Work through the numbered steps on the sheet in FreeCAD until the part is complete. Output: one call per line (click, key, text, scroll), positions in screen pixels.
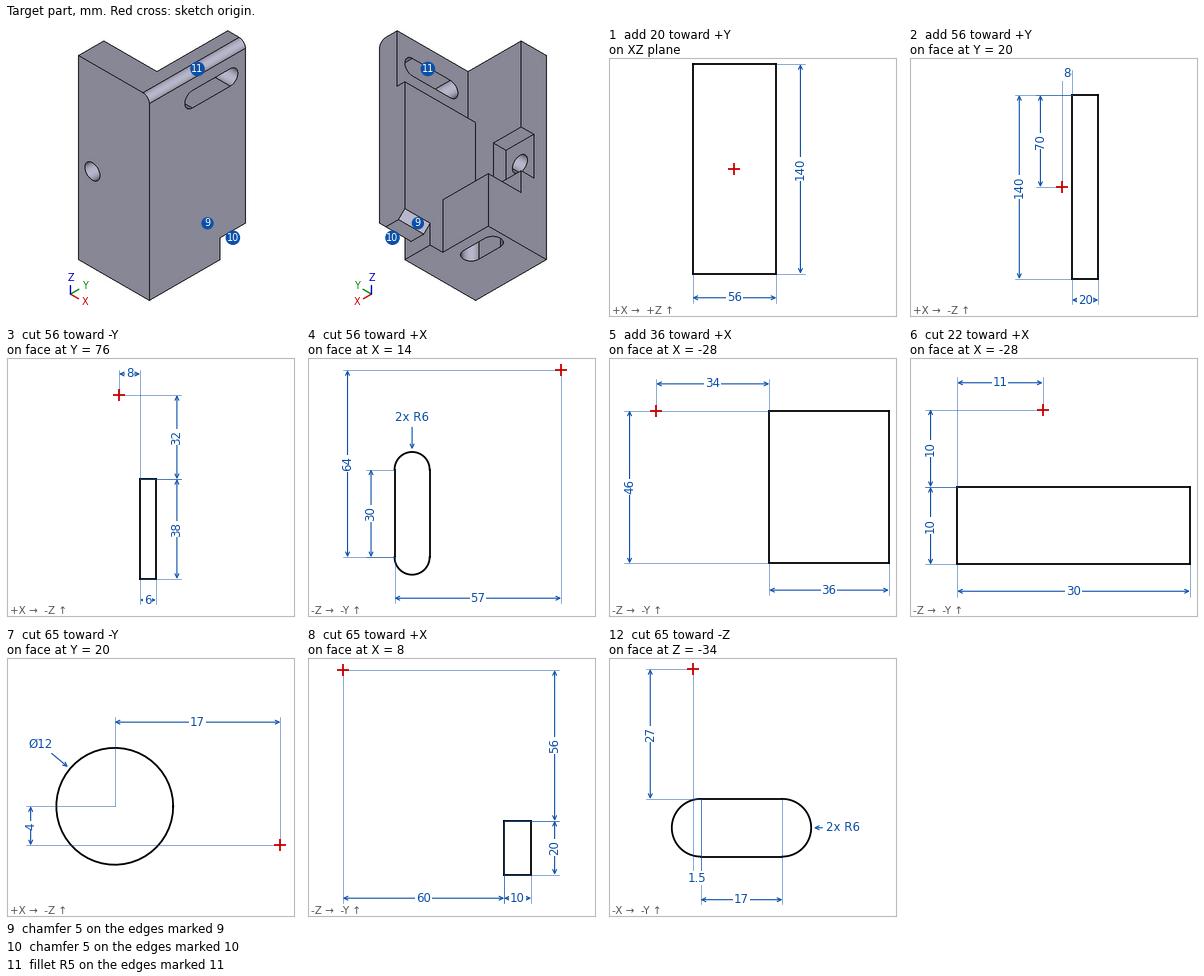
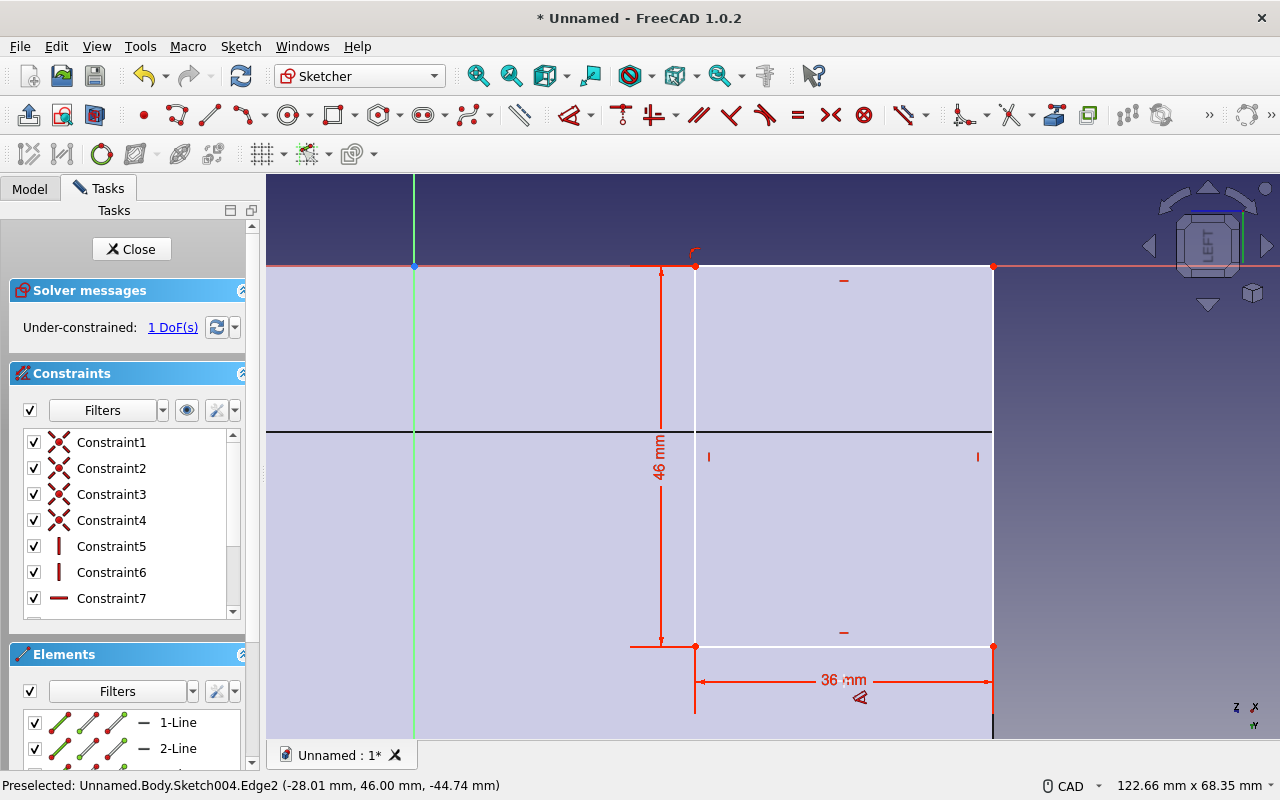
click(695, 266)
click(555, 232)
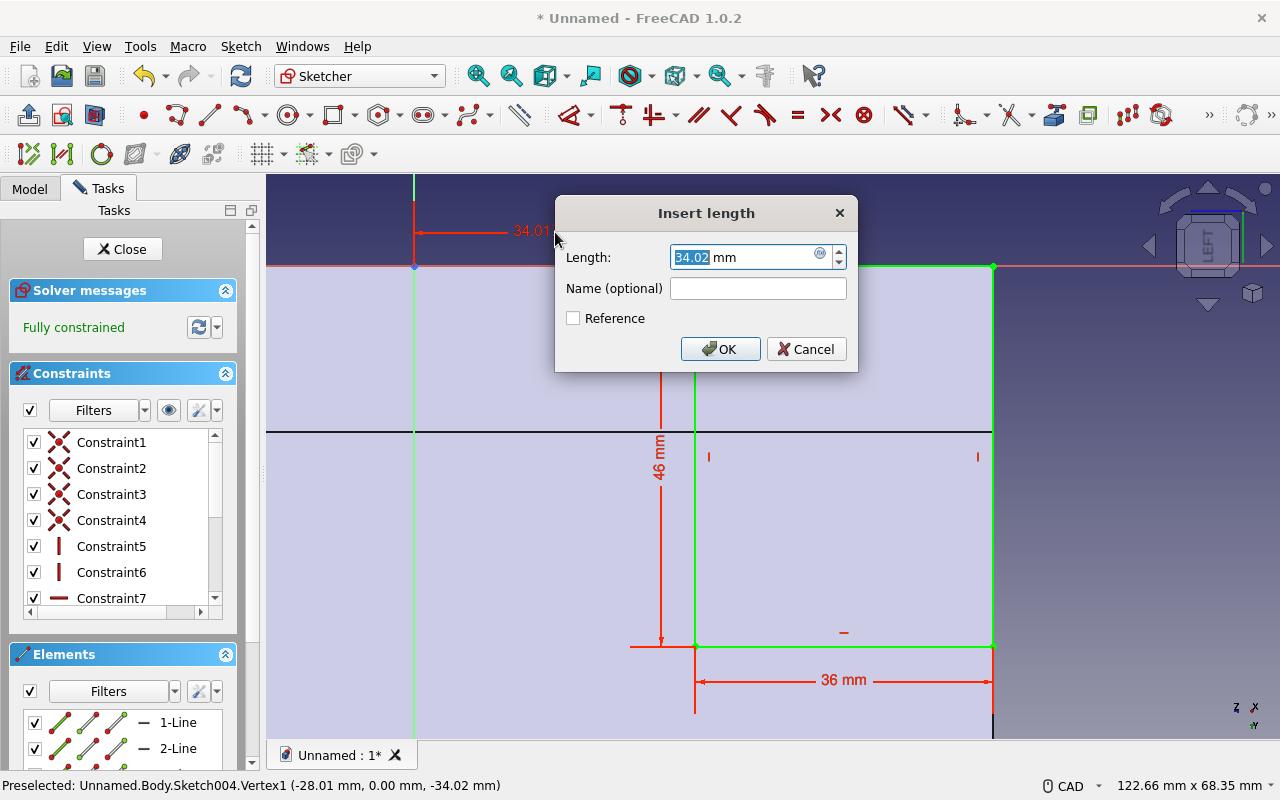
text(34)
key(Return)
key(Escape)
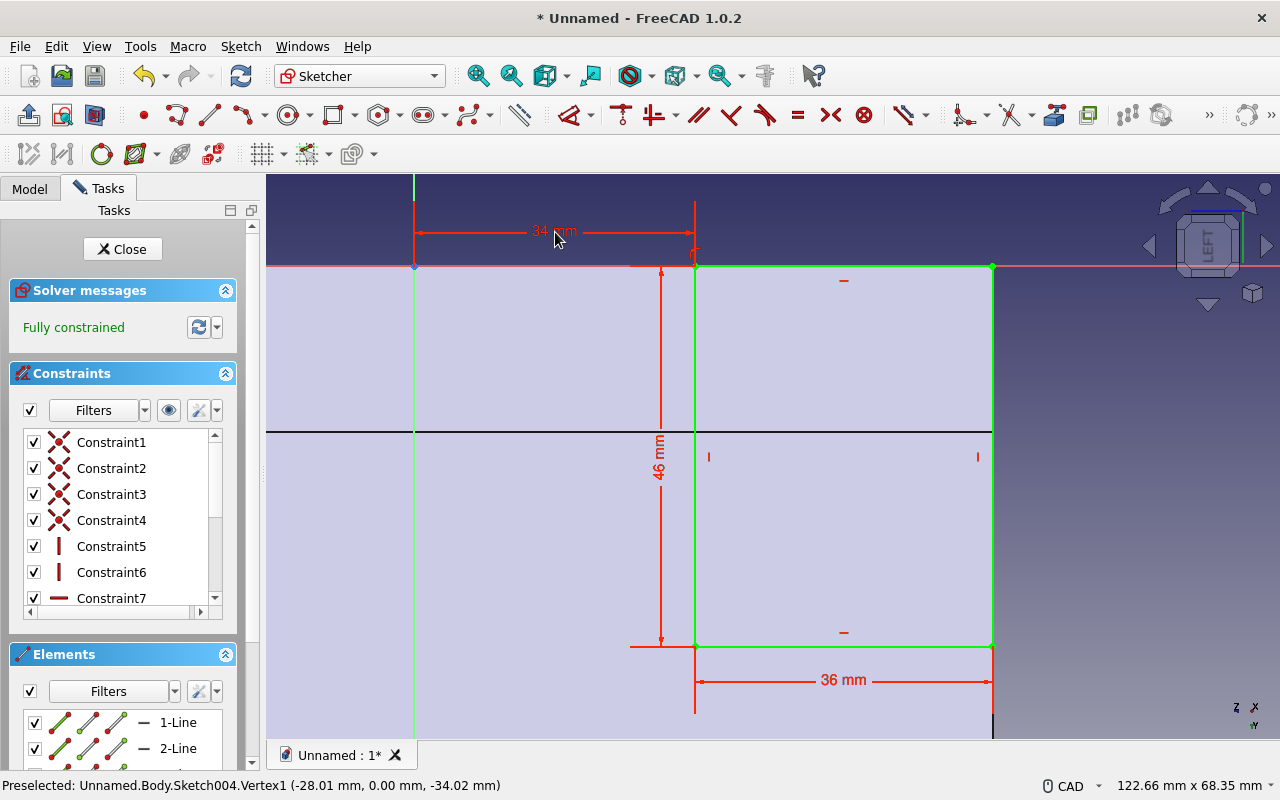
click(123, 249)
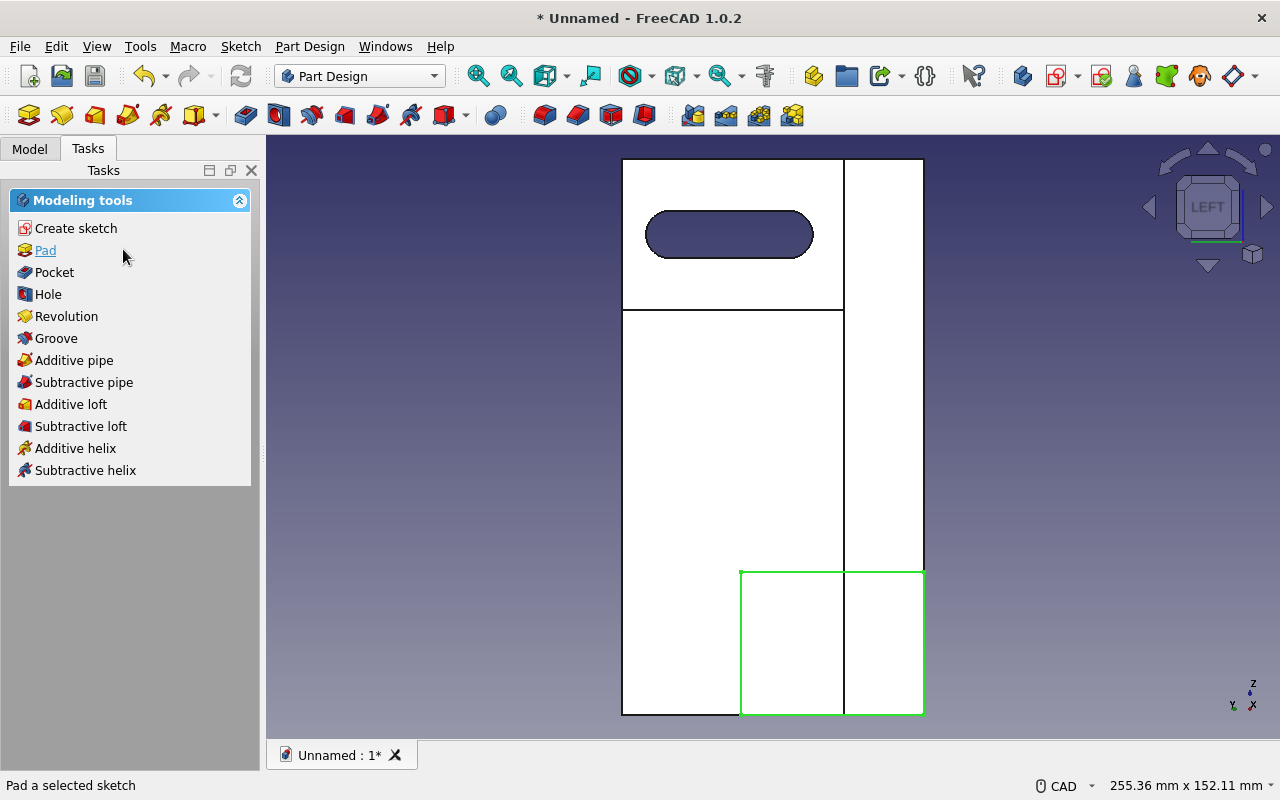
click(29, 116)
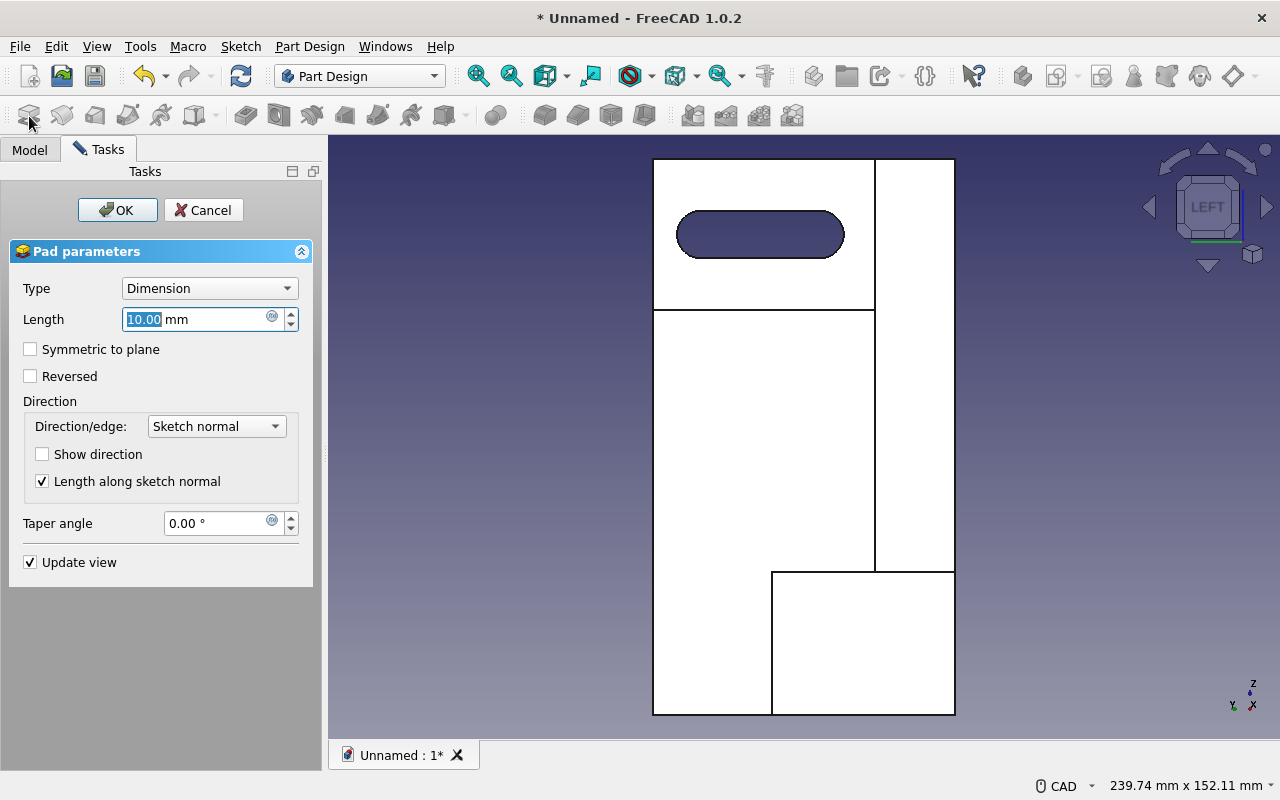
text(36)
key(Tab)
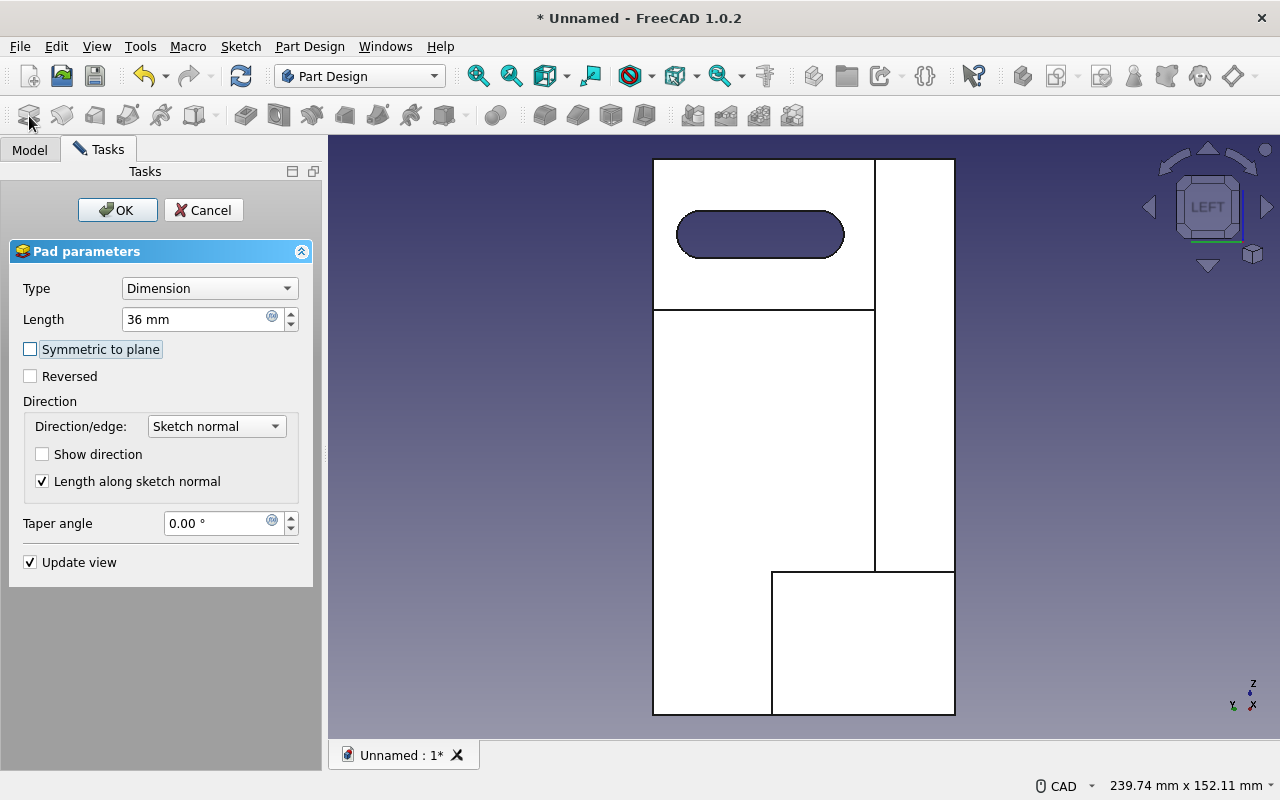
click(31, 376)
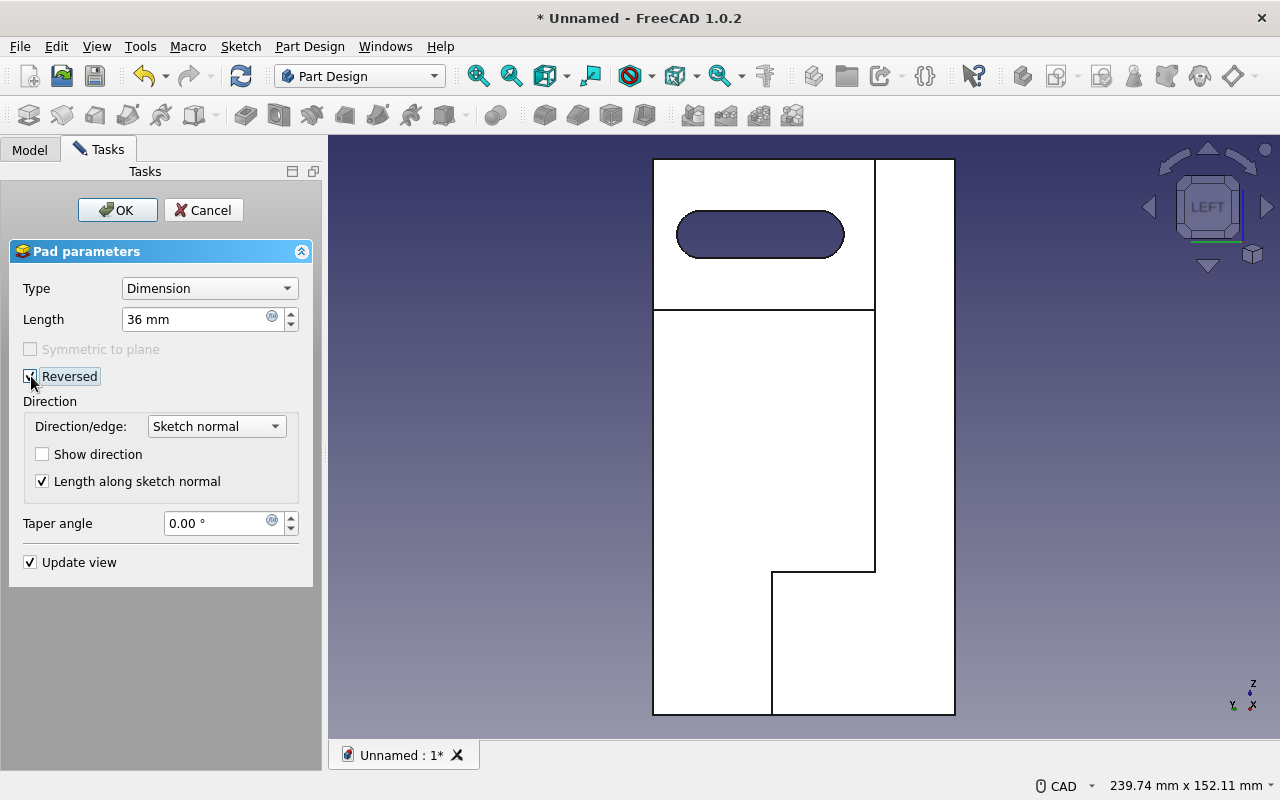
click(118, 210)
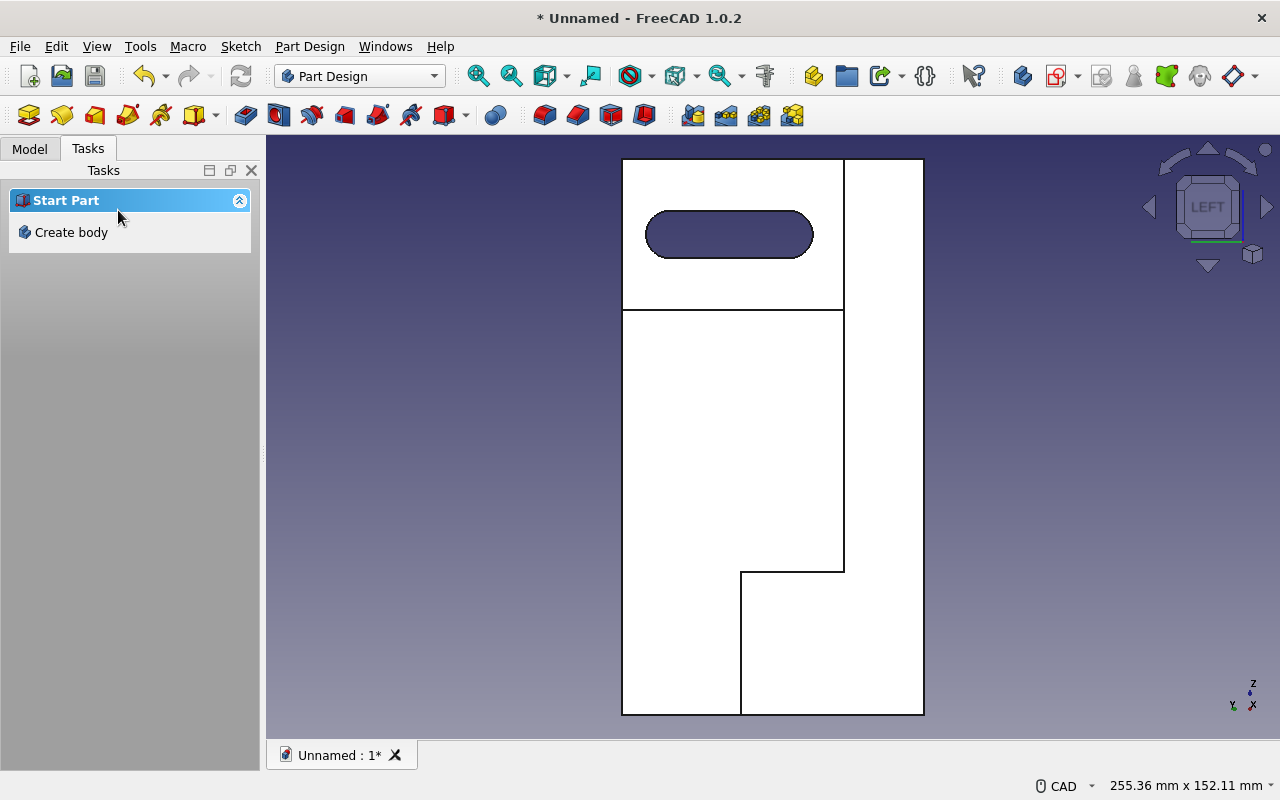
click(806, 674)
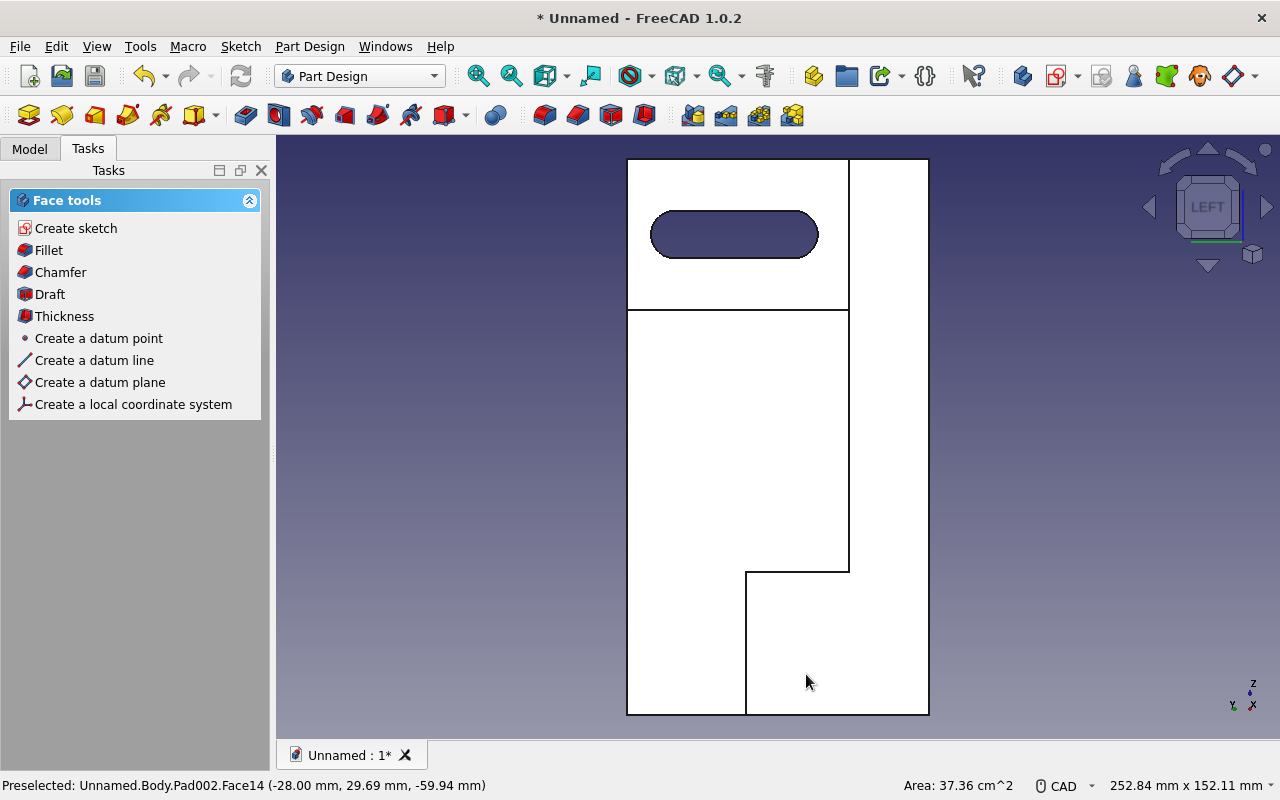
click(1056, 76)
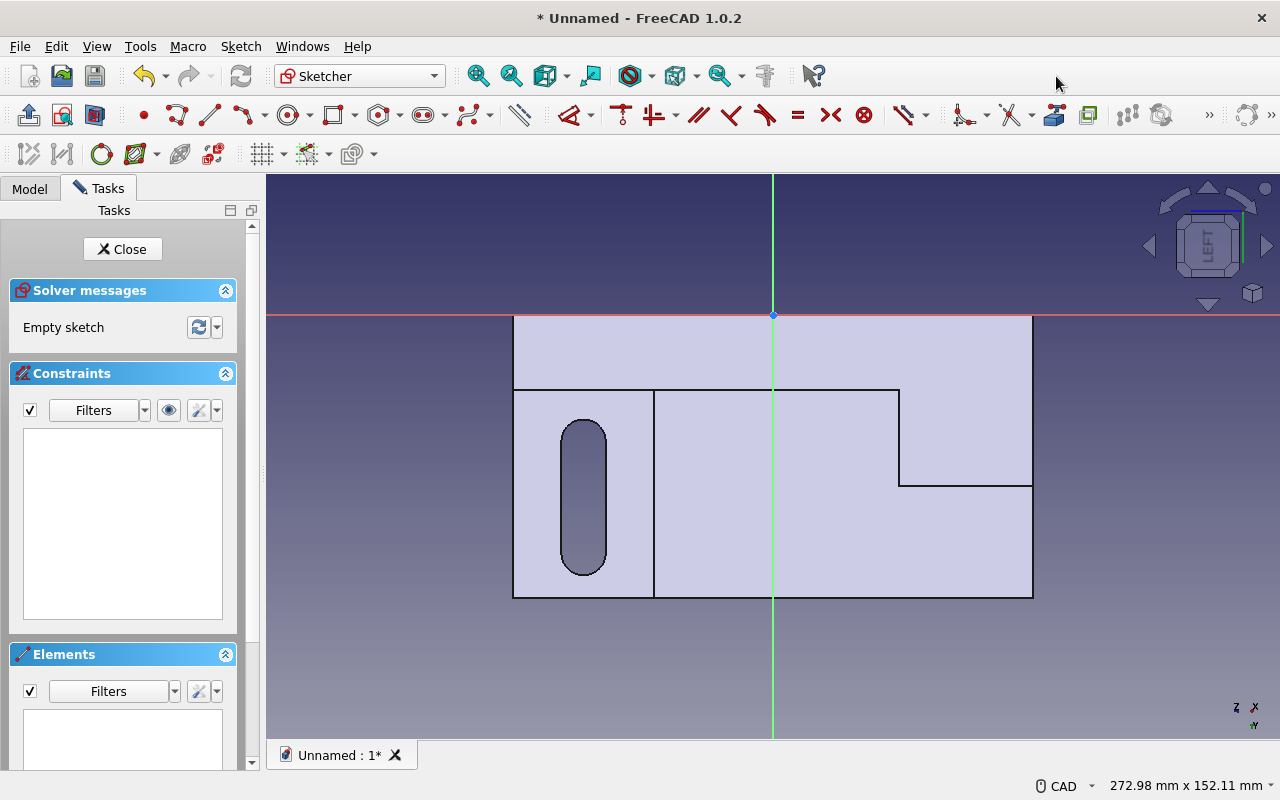
scroll(809, 326, up, 8)